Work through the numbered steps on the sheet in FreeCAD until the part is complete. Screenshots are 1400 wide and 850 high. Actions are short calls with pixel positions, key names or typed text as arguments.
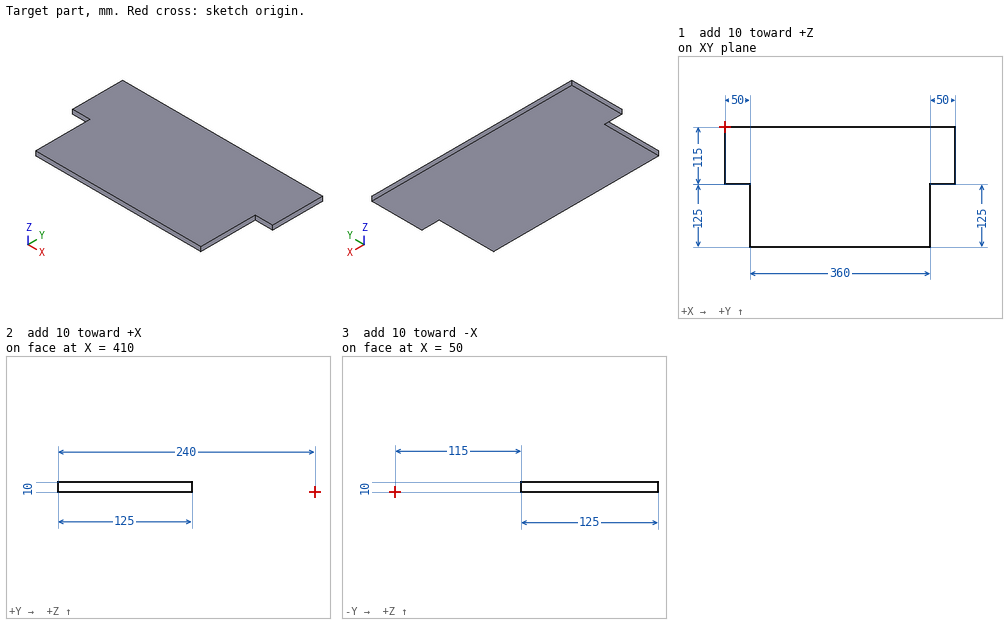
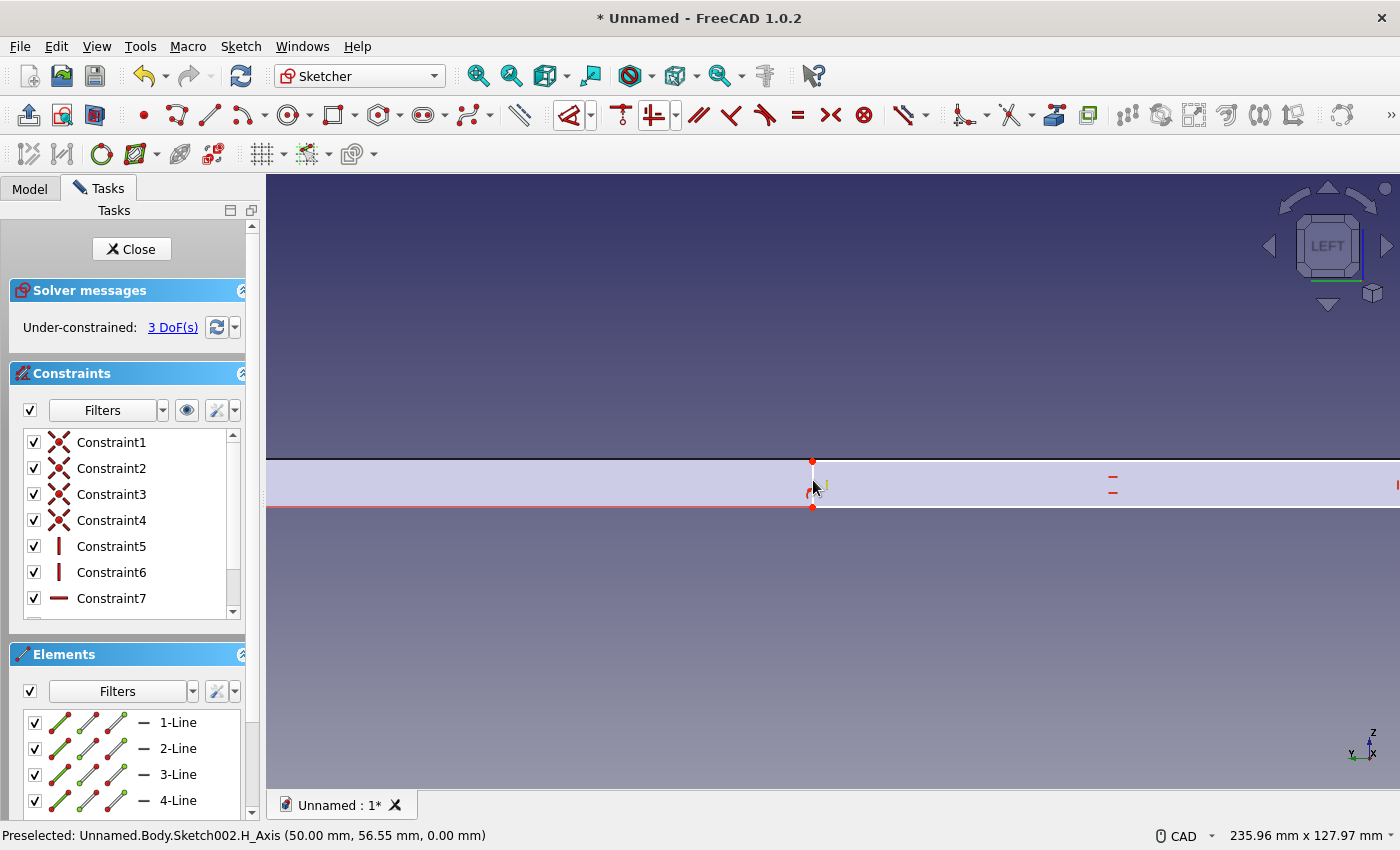
click(813, 480)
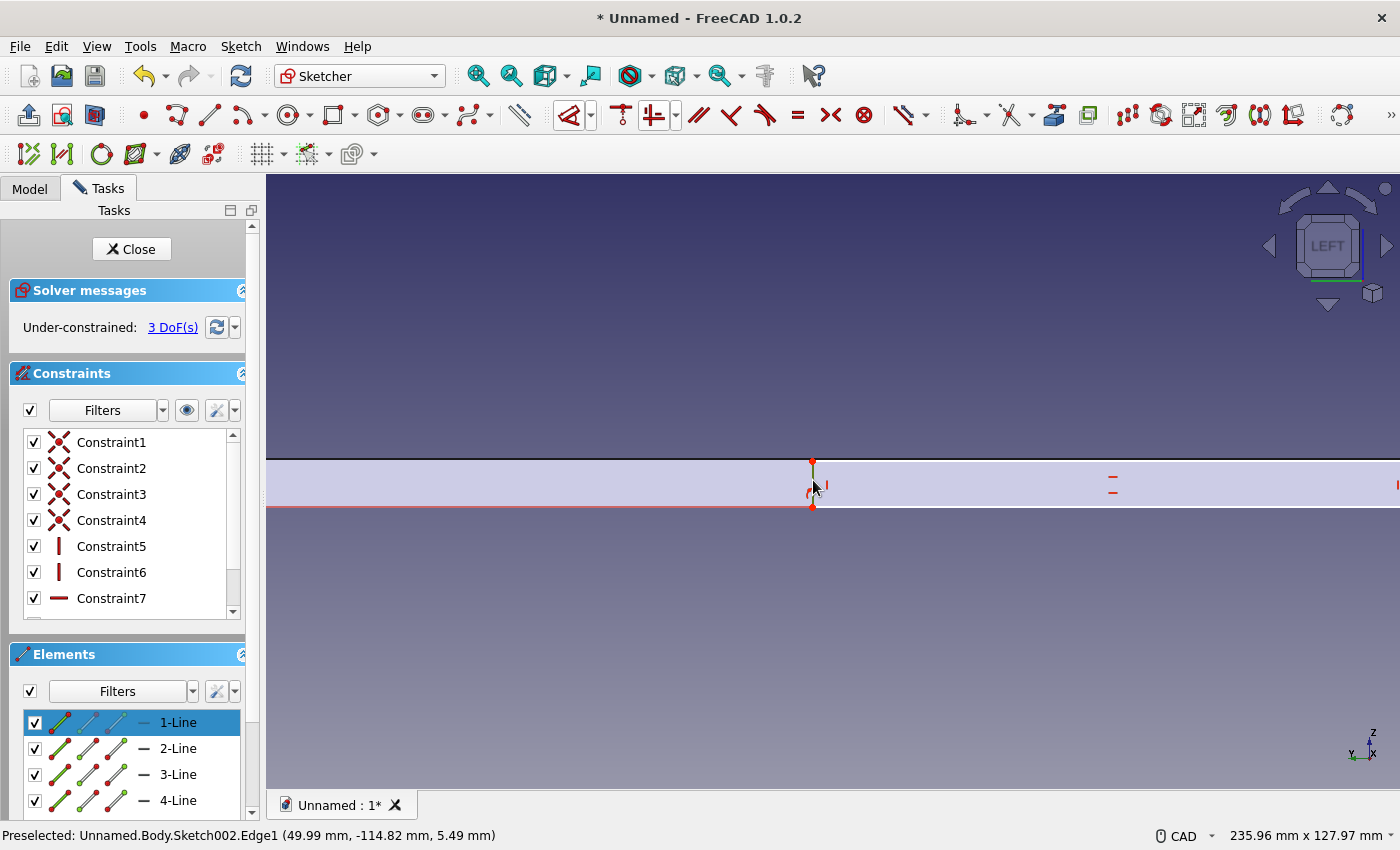
click(590, 116)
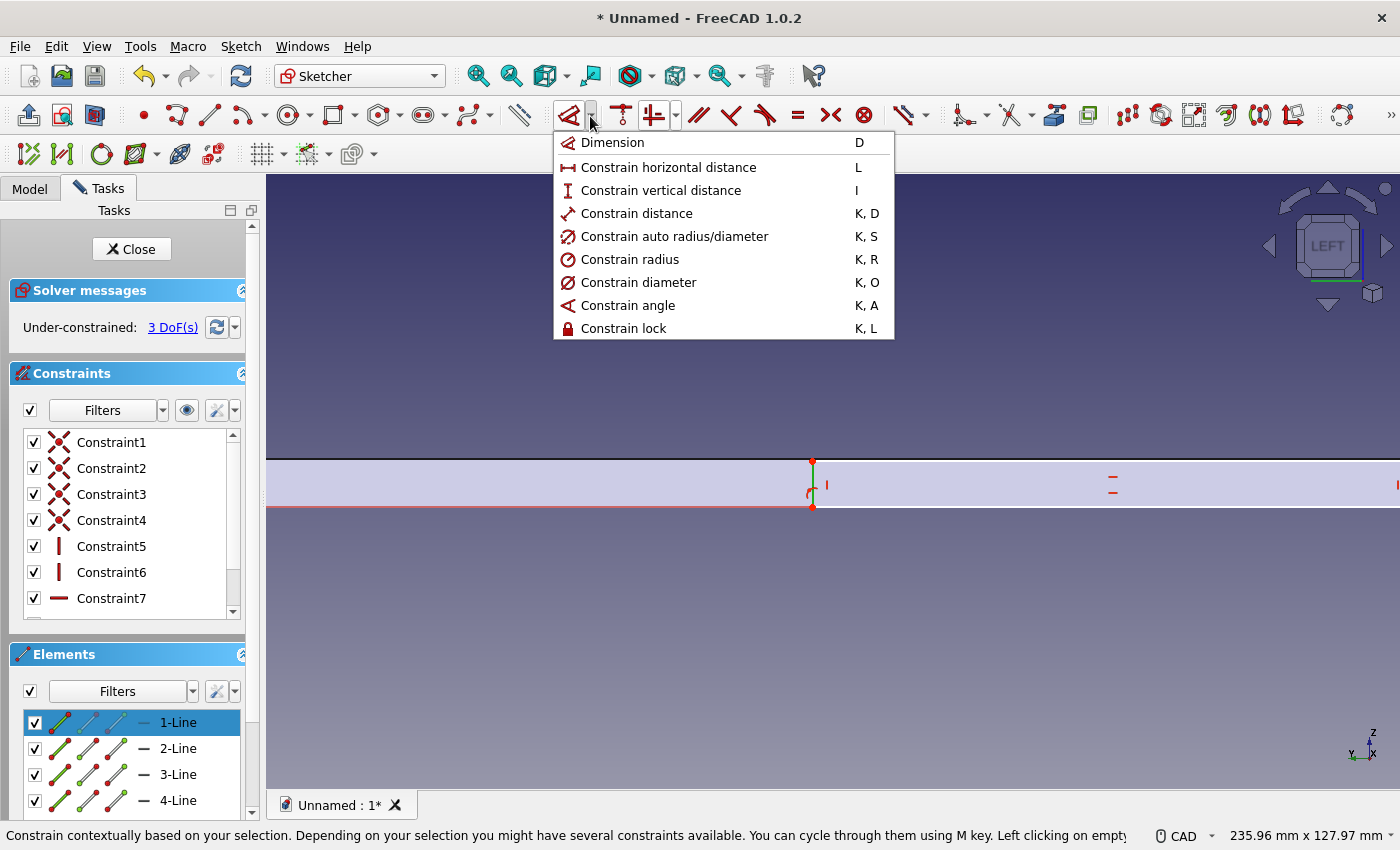
click(724, 190)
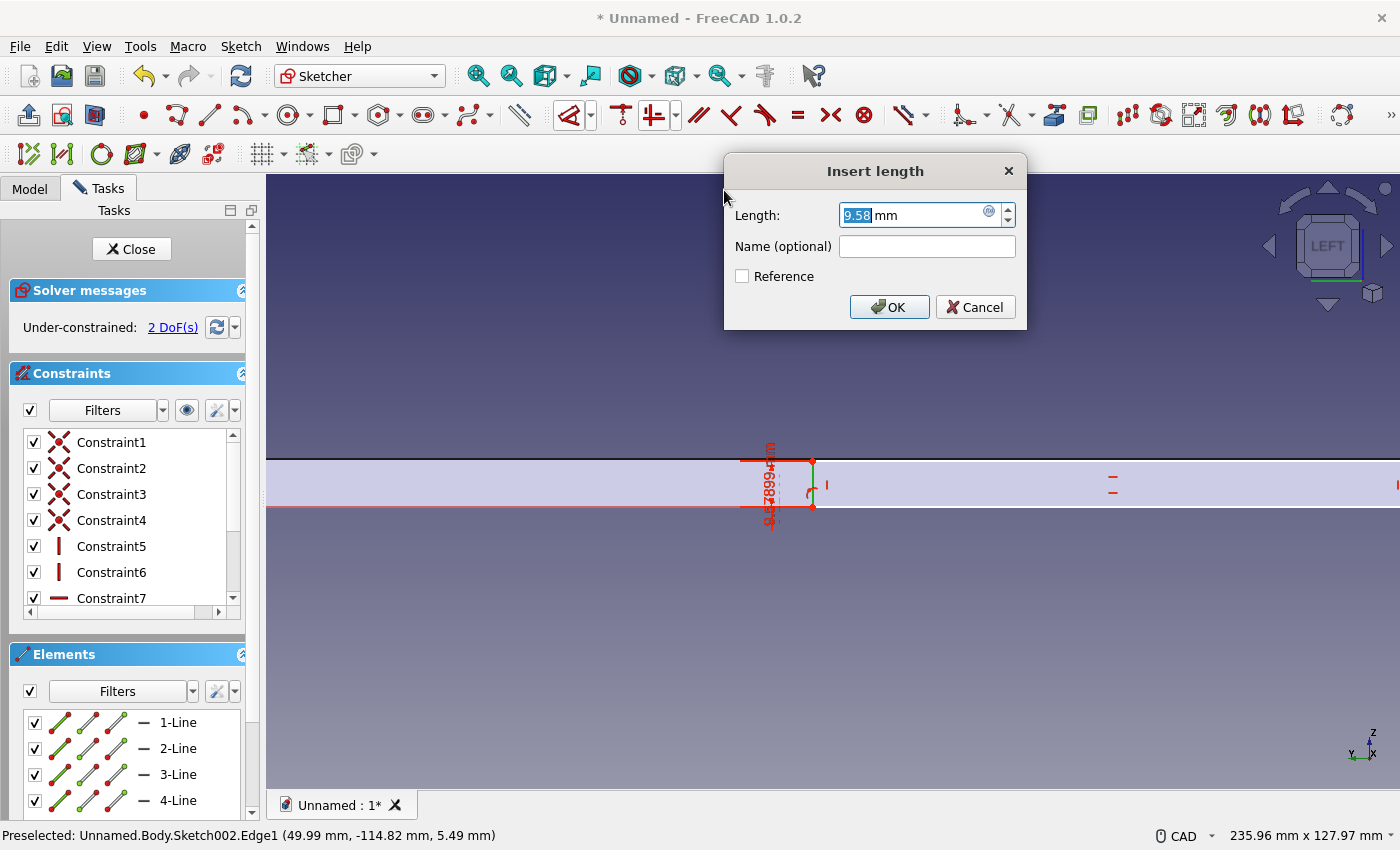
text(10)
key(Return)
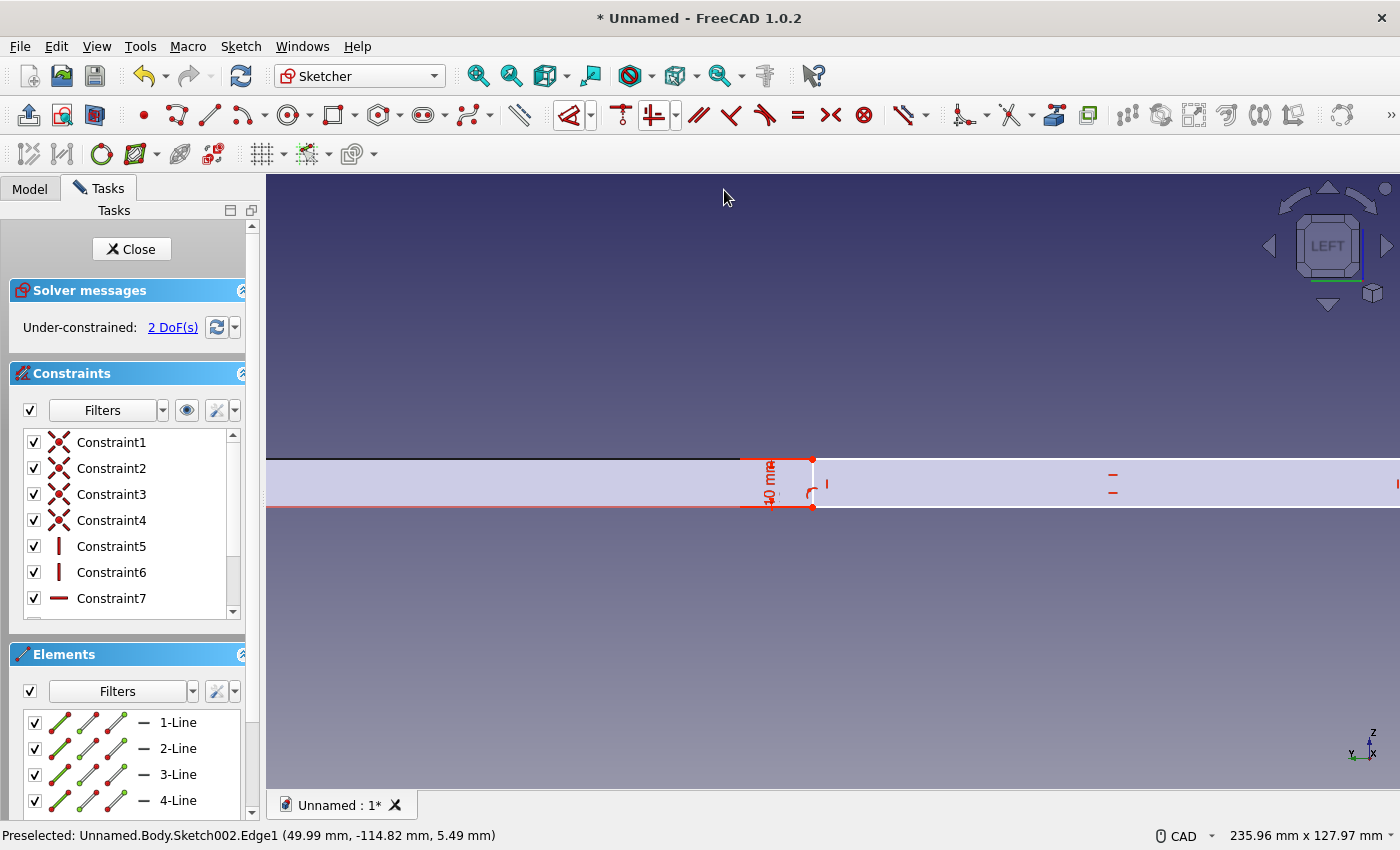
click(993, 507)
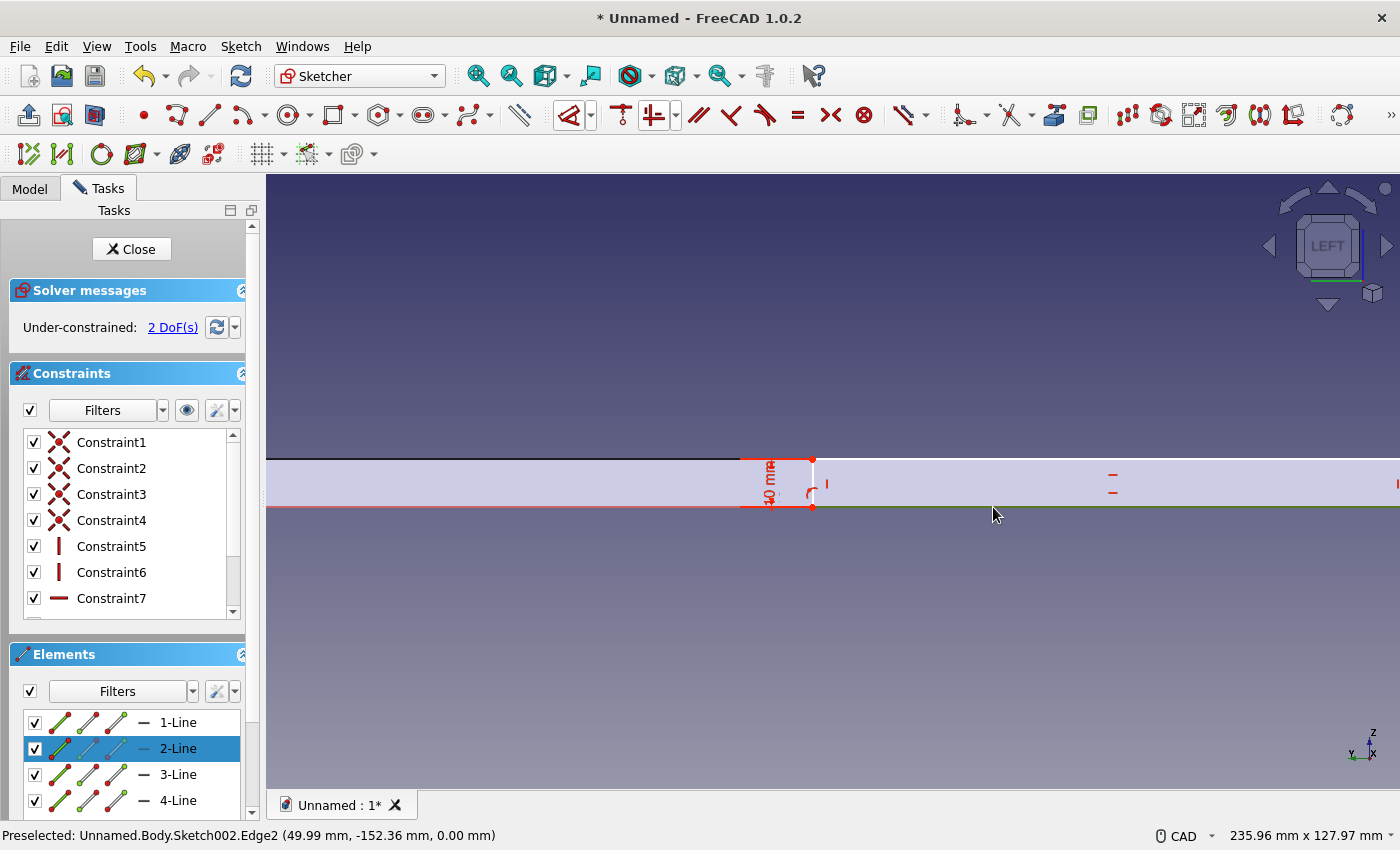
key(l)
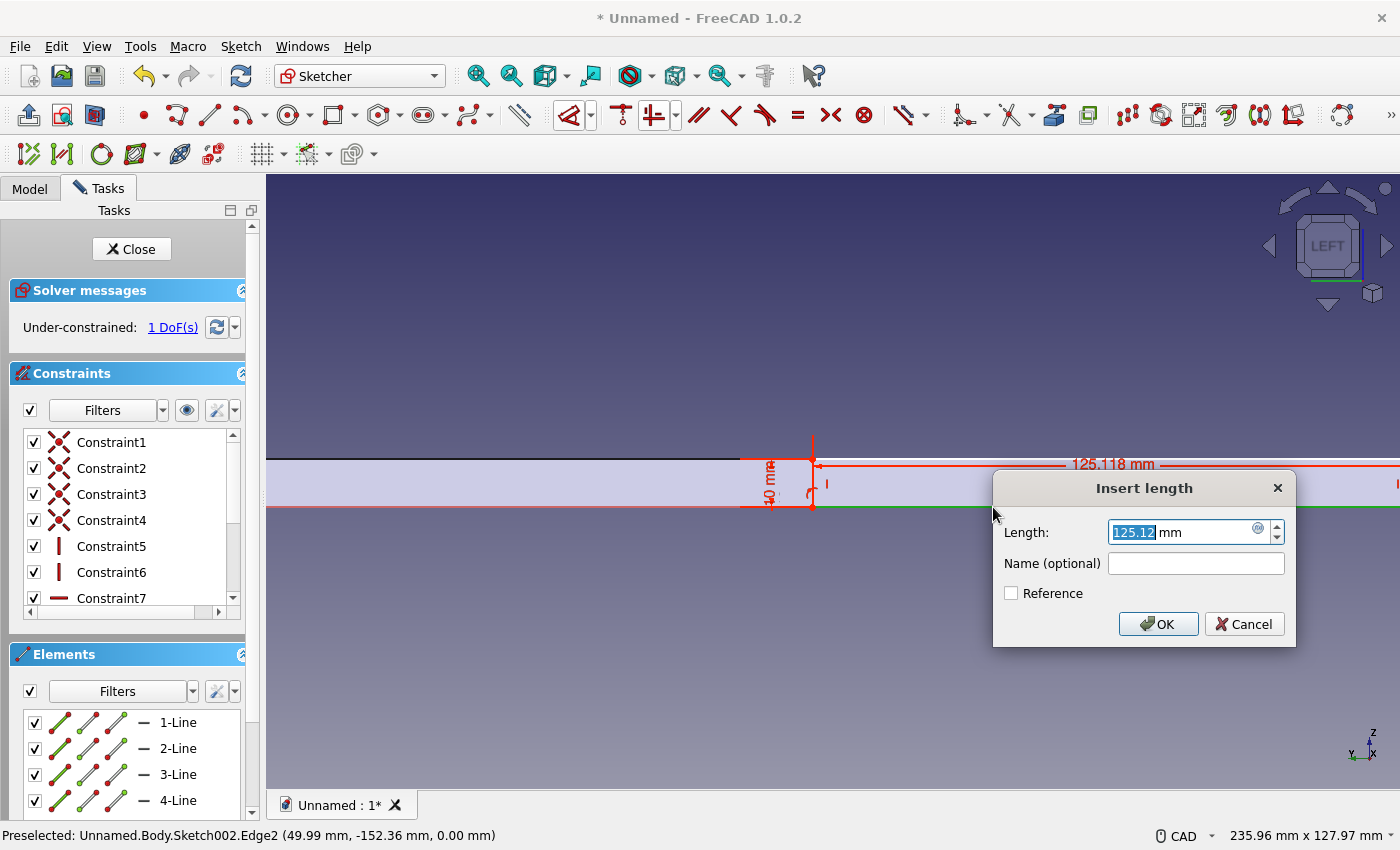
text(125)
key(Return)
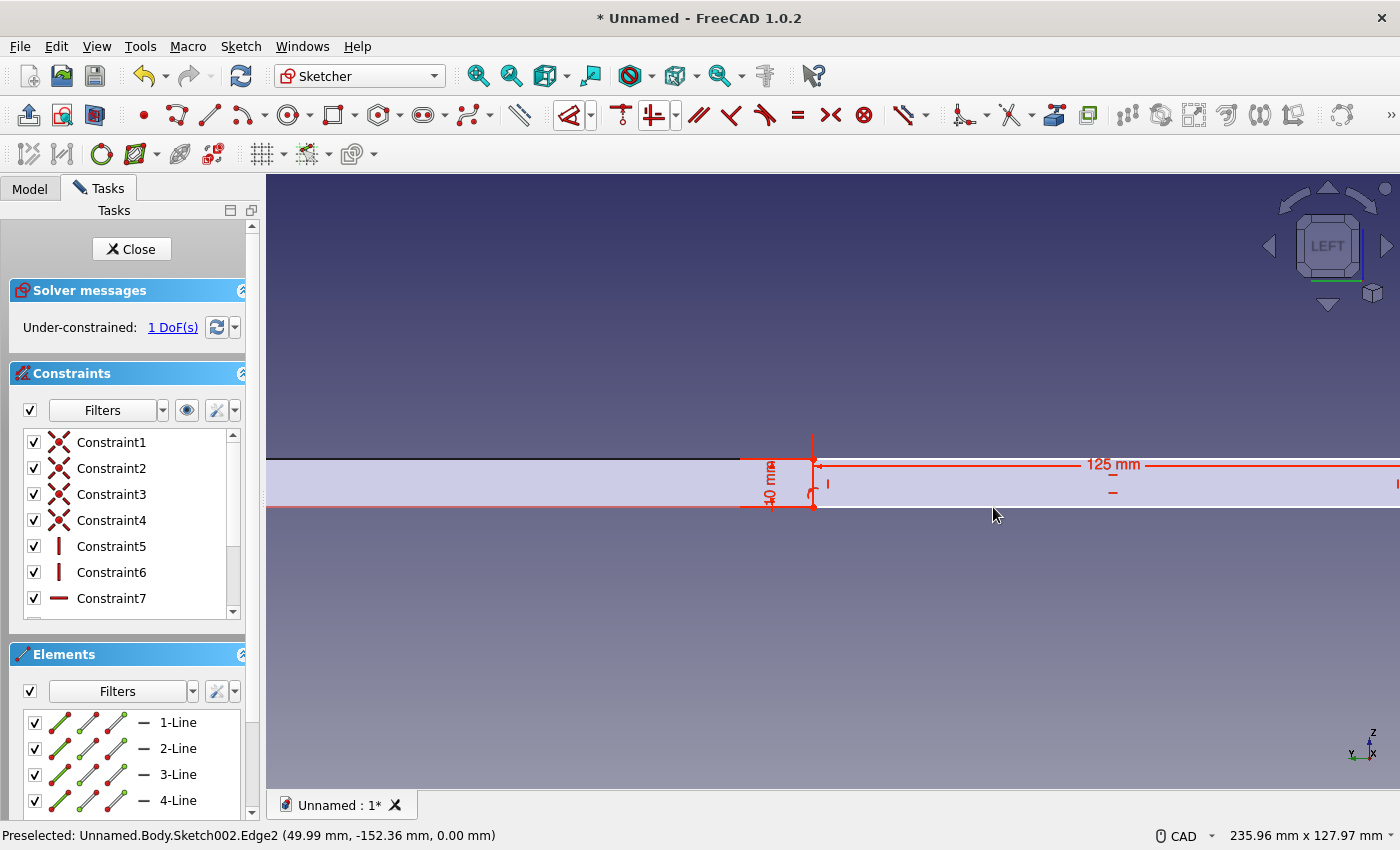
click(813, 459)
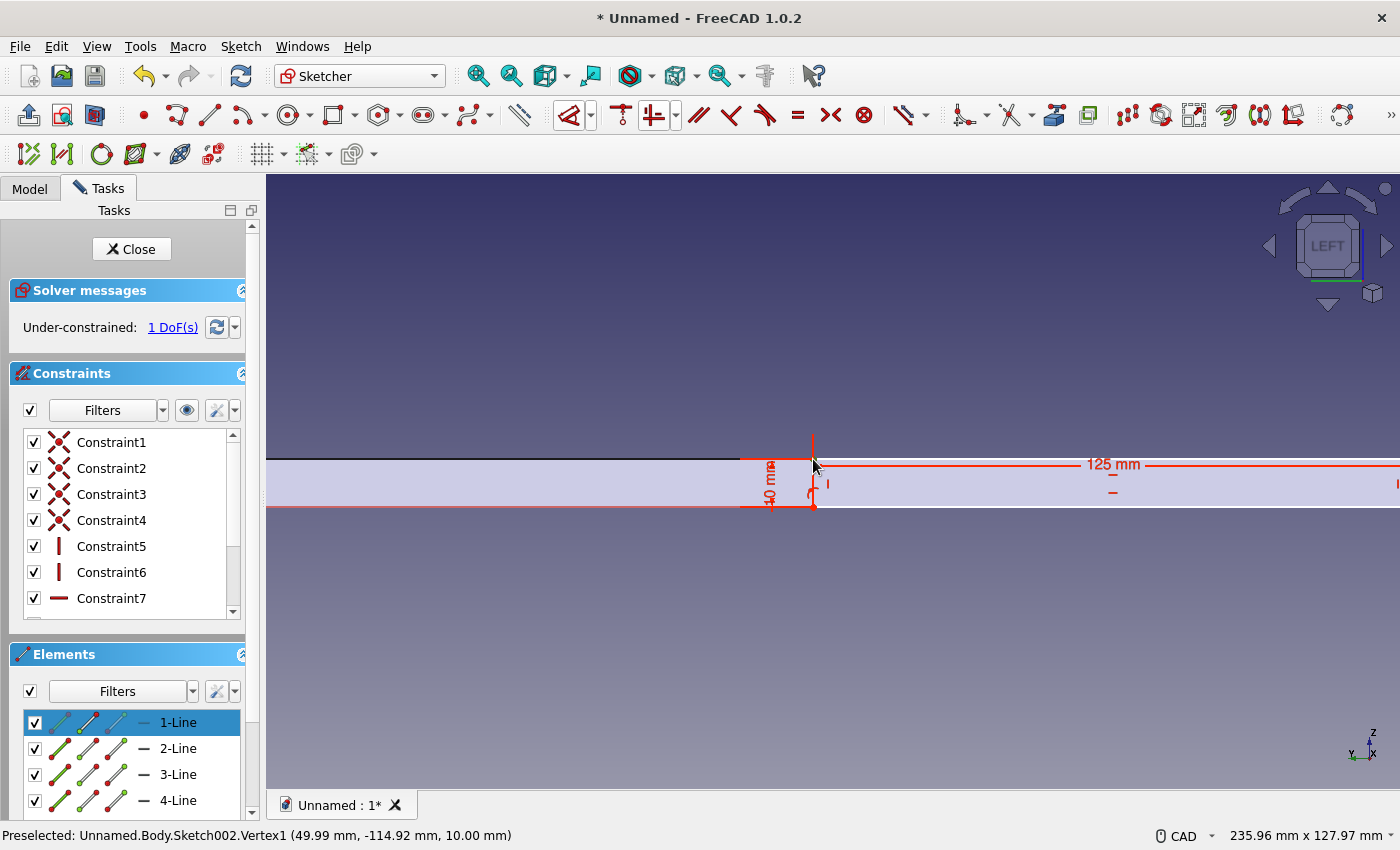
click(590, 116)